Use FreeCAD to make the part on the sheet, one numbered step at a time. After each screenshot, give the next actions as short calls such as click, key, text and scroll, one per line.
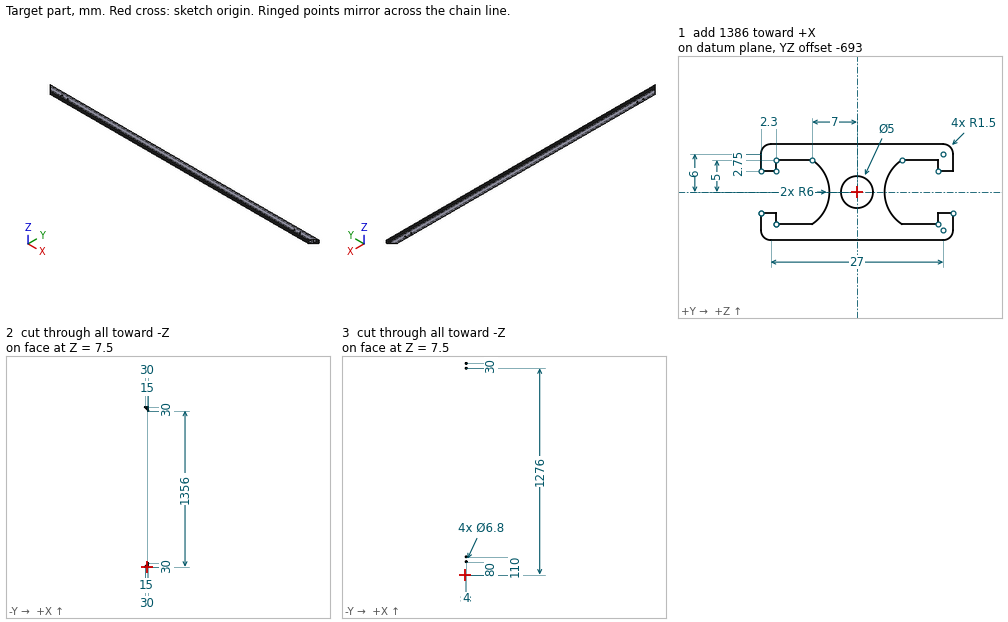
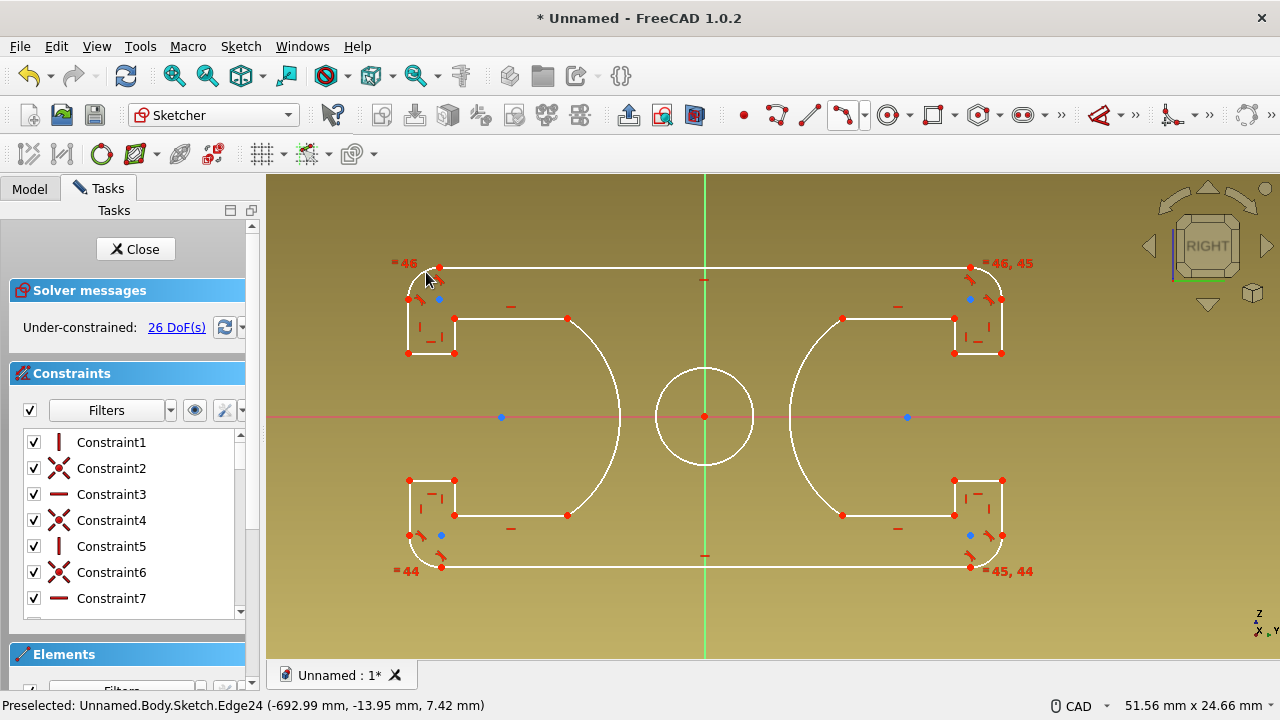
click(611, 463)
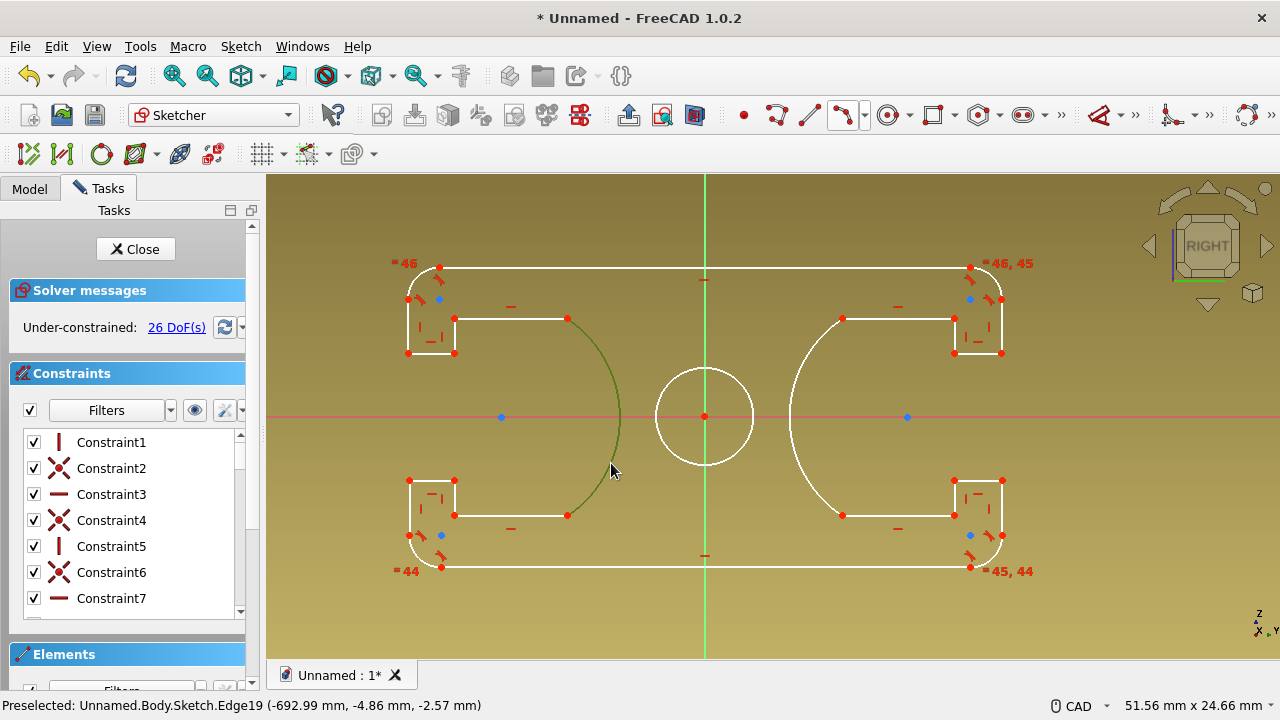
click(799, 372)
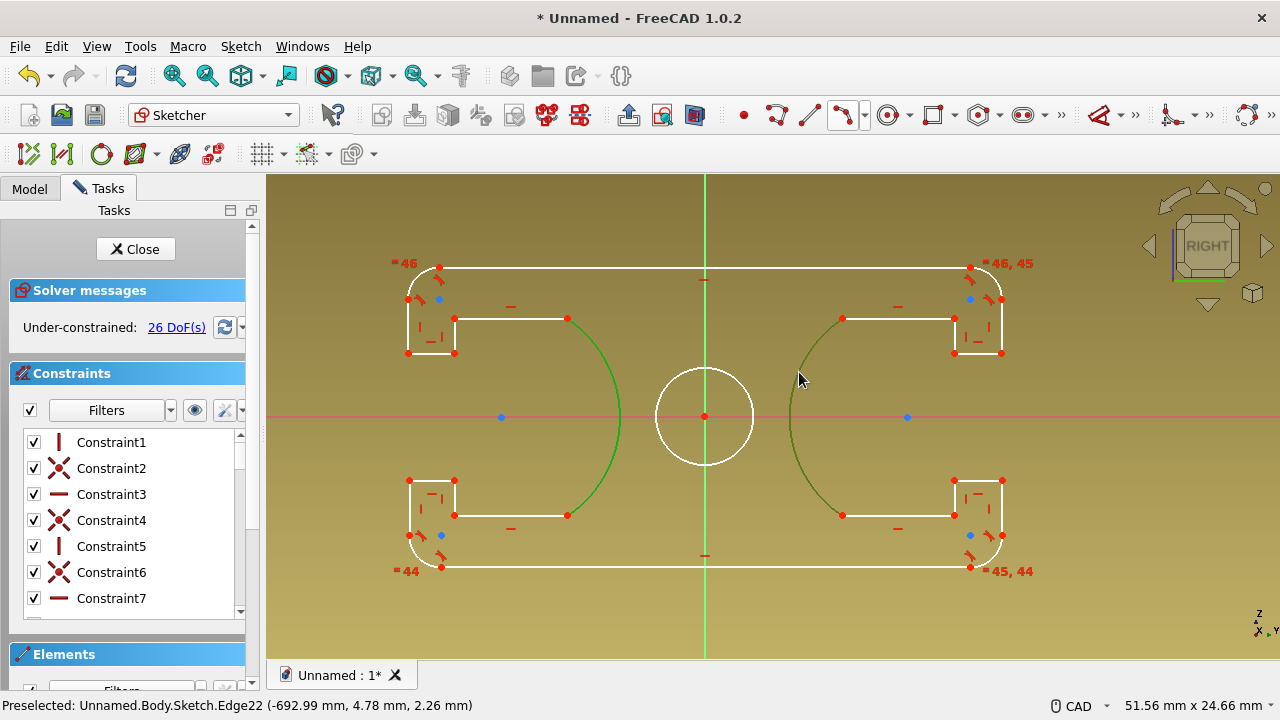
key(e)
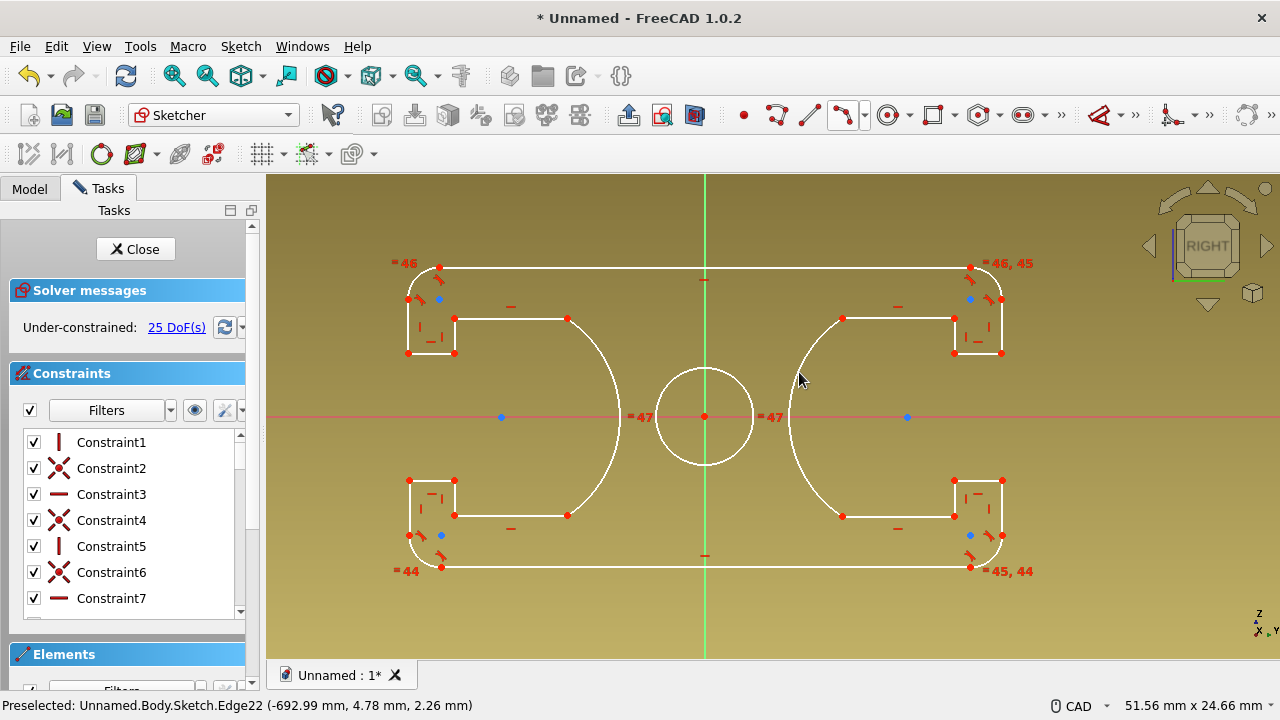
click(501, 417)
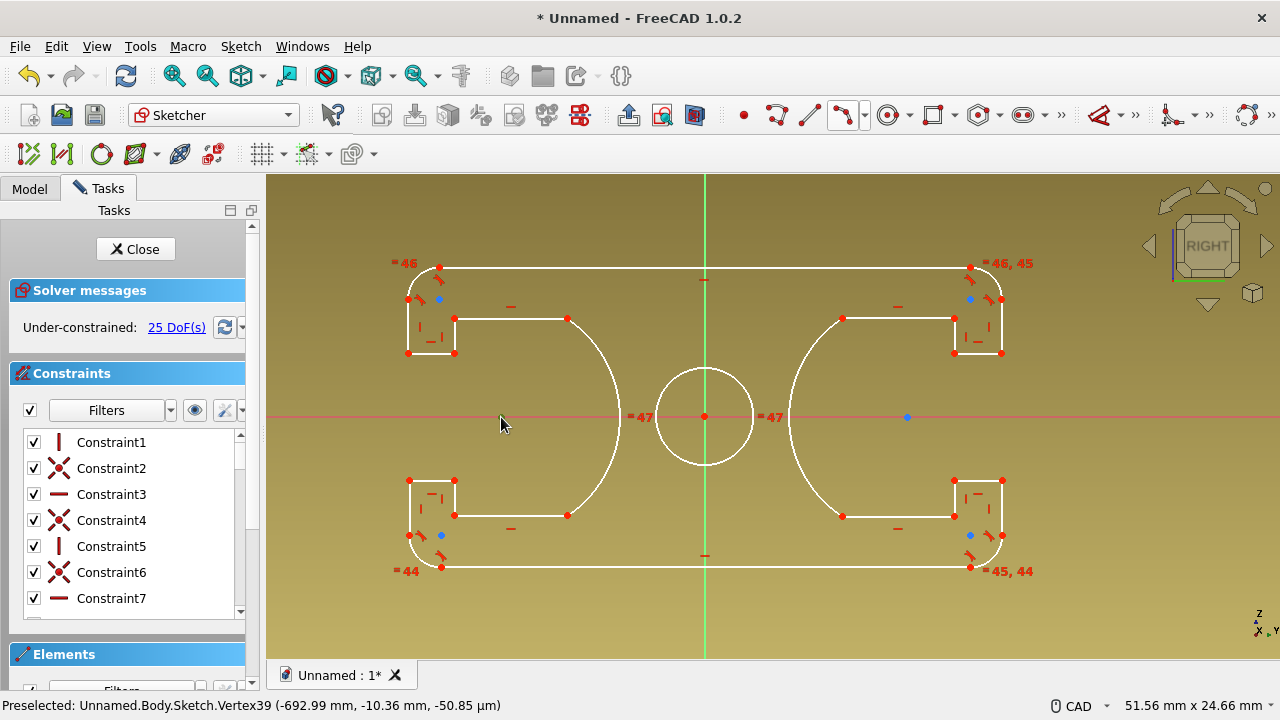
click(353, 416)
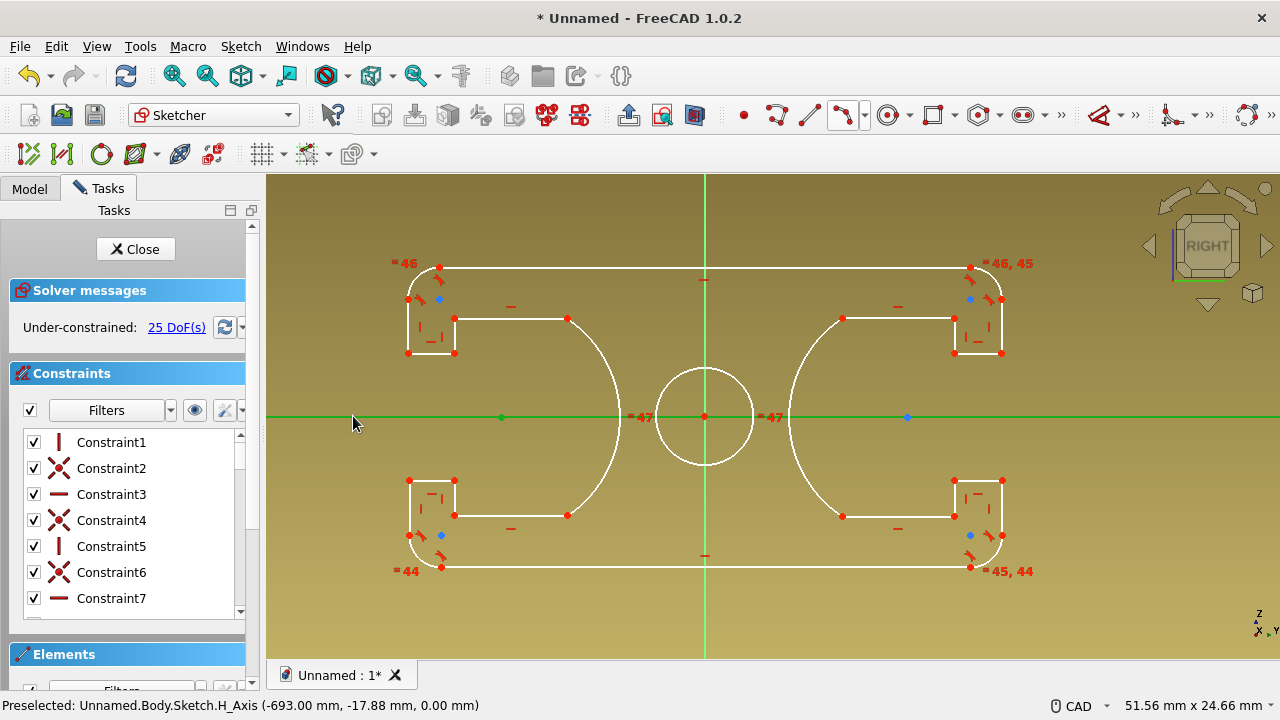
key(c)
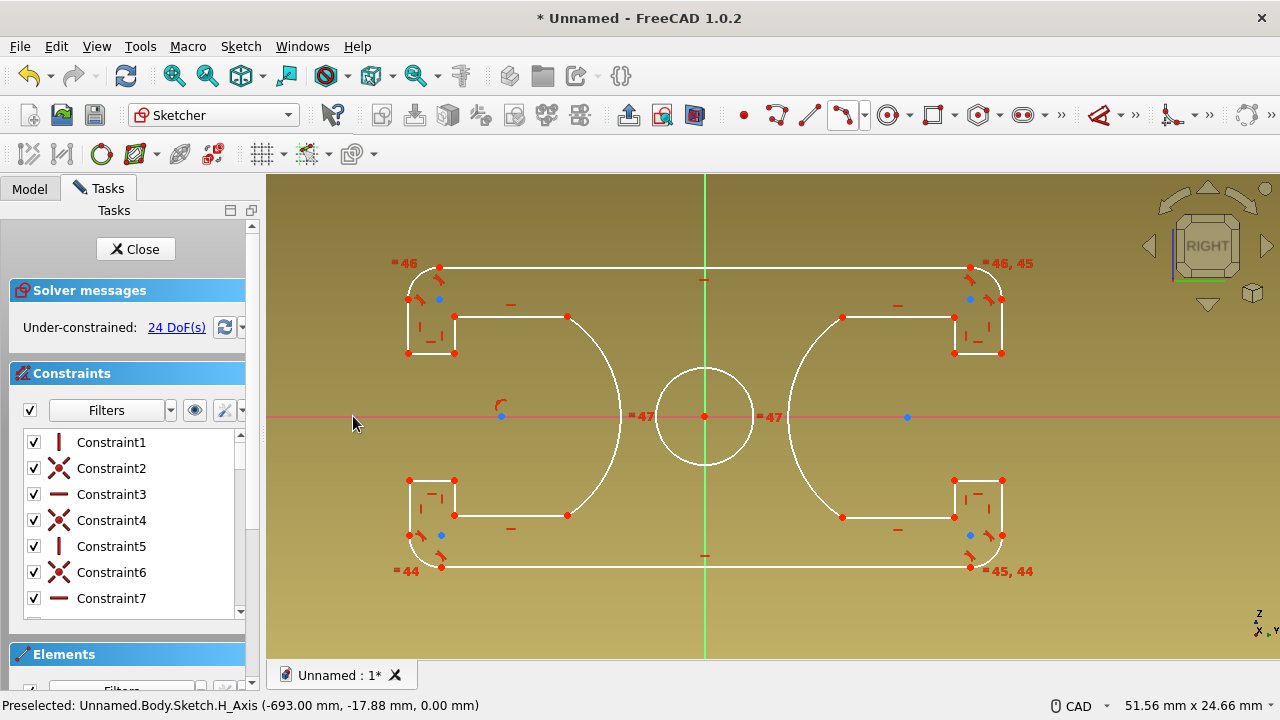
click(908, 417)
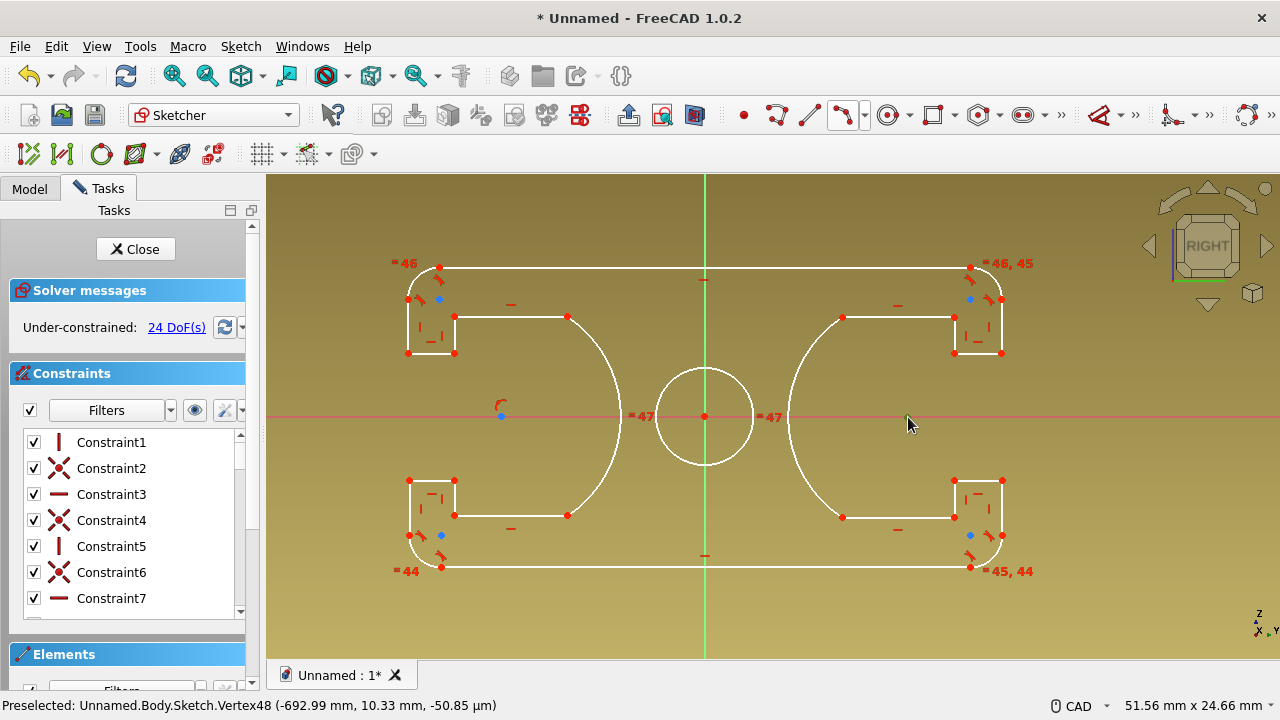
click(353, 416)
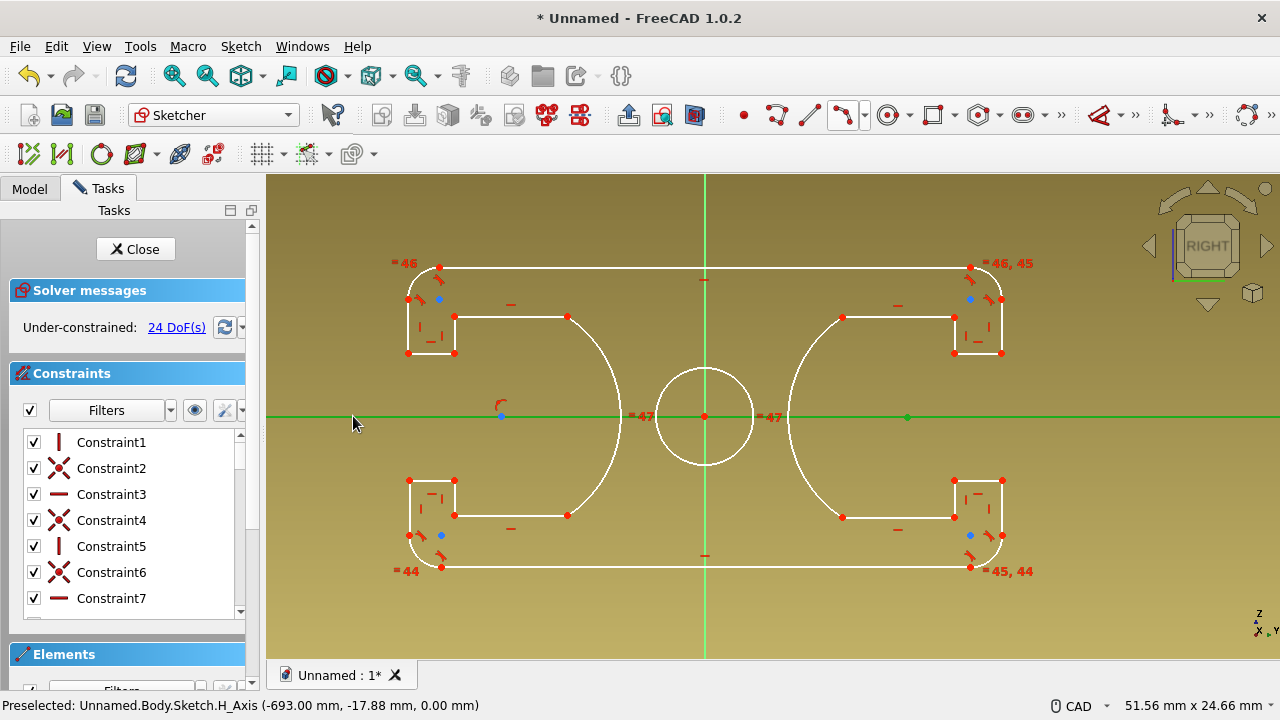
key(c)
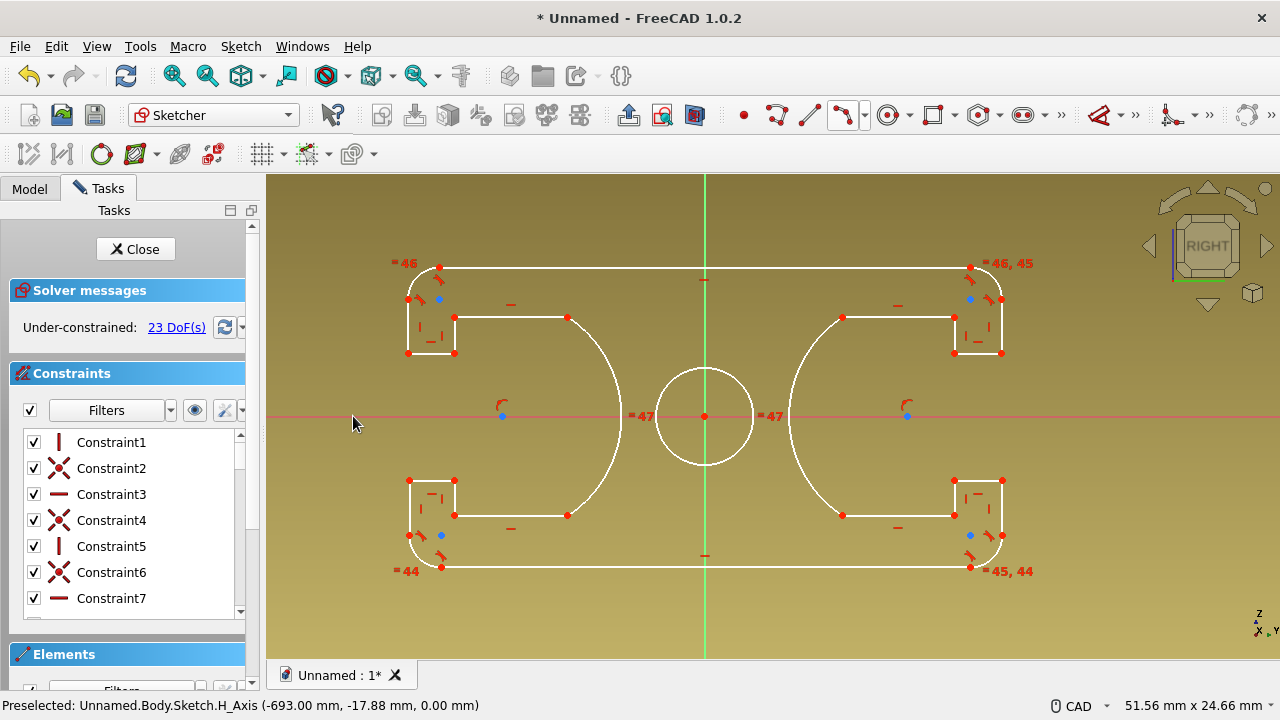
click(971, 536)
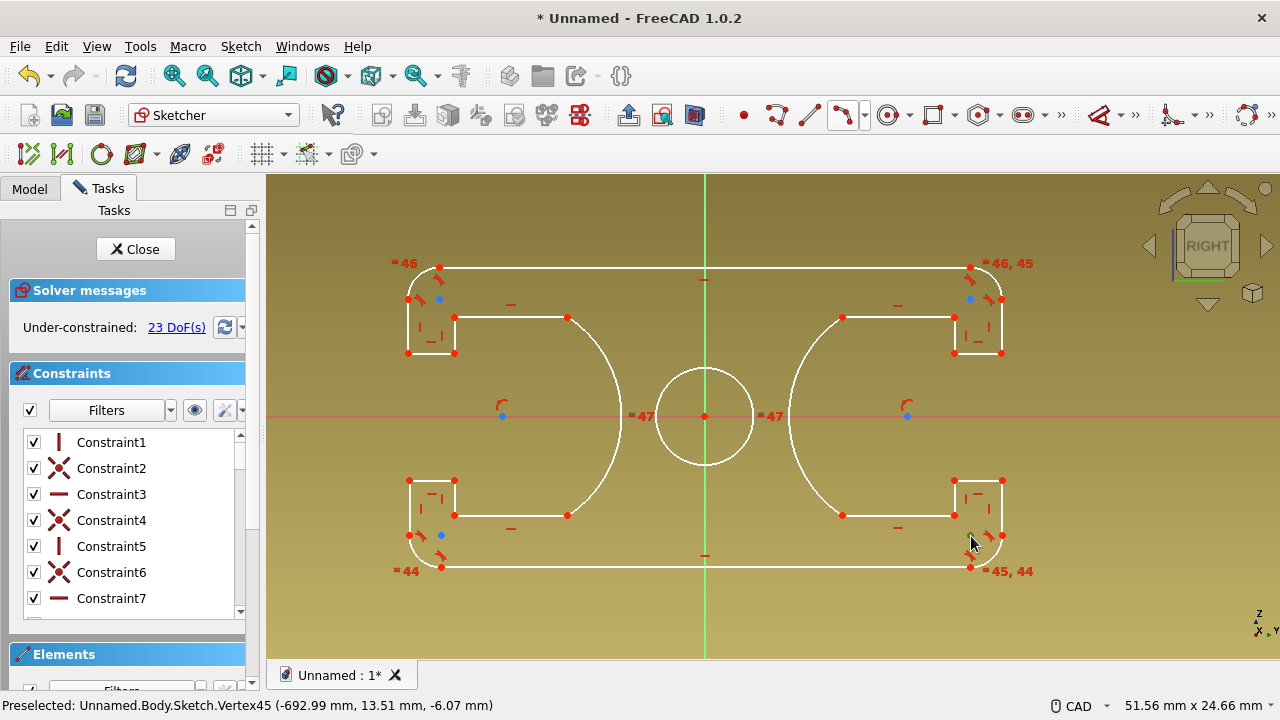
click(970, 299)